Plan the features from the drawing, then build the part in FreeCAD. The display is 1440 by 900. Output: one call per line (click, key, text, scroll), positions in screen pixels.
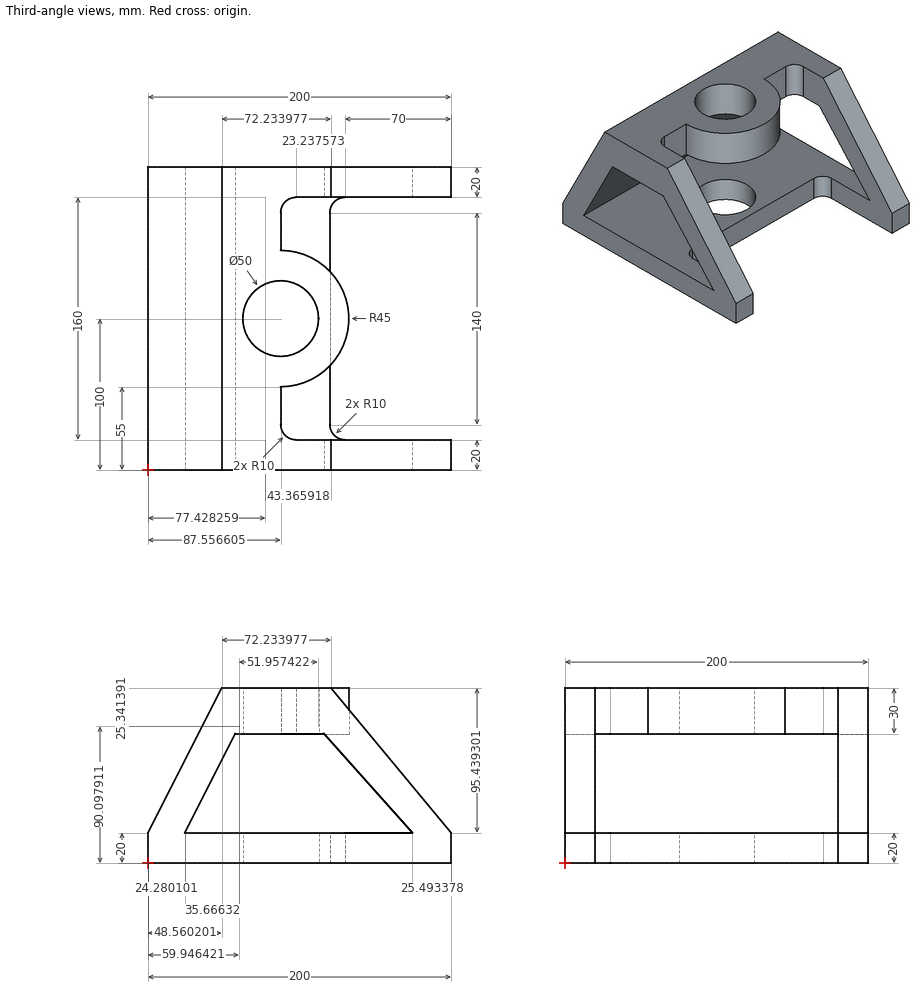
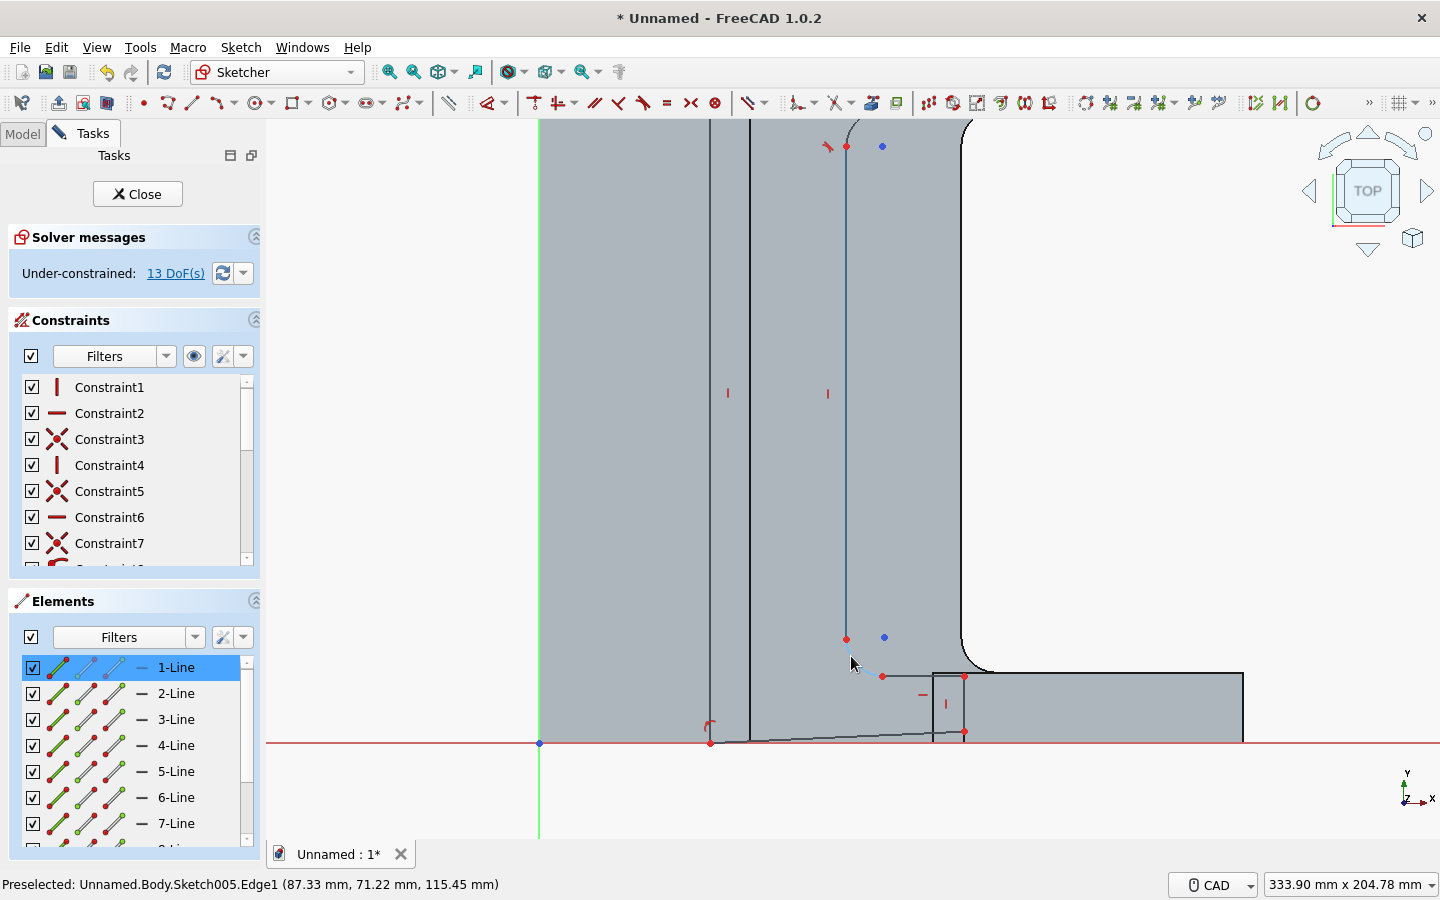
click(851, 655)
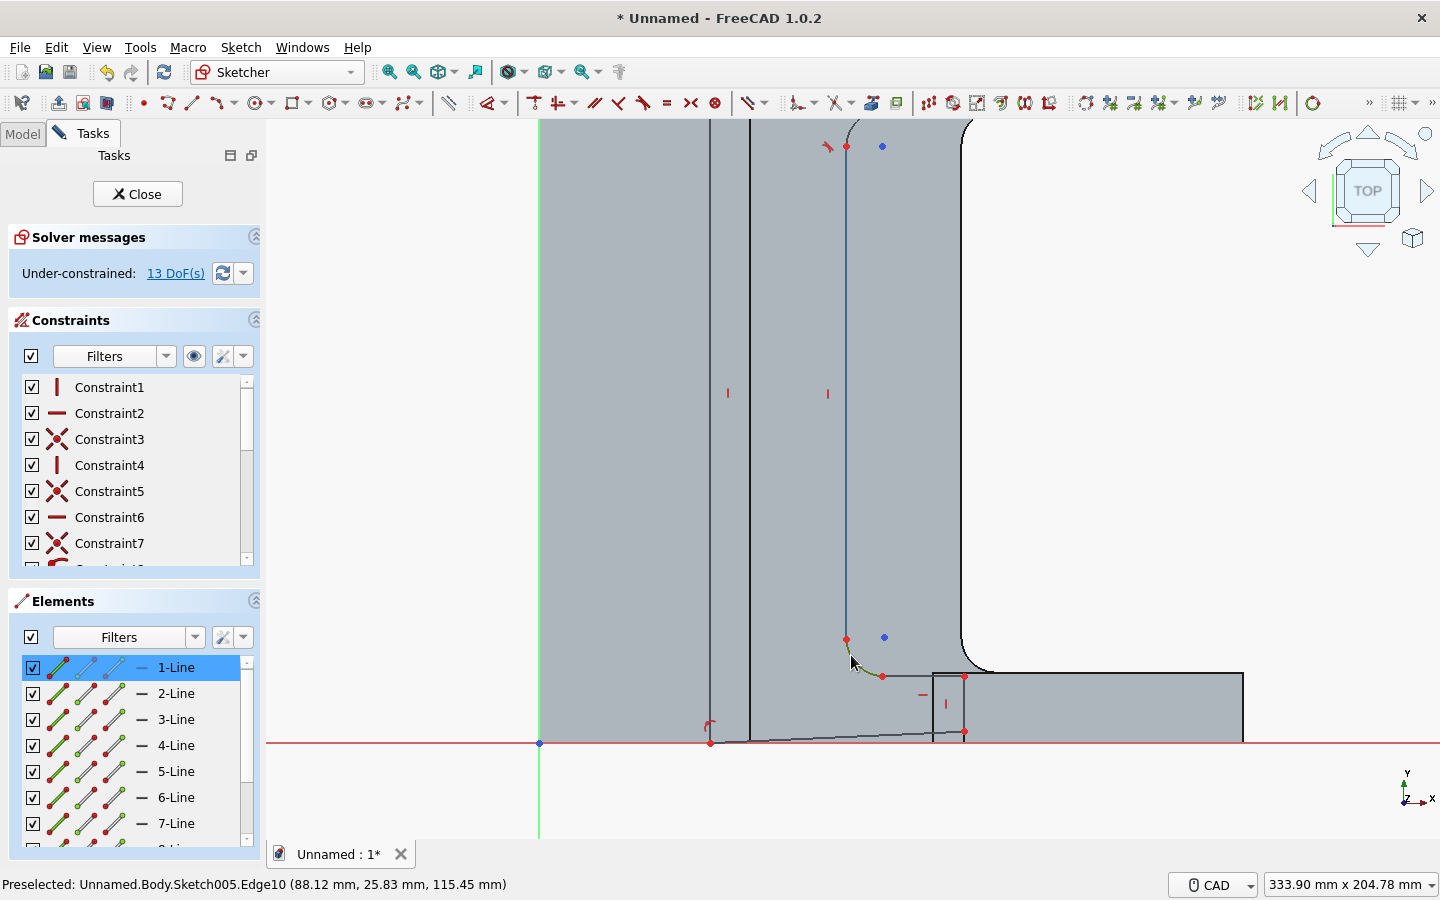
click(644, 104)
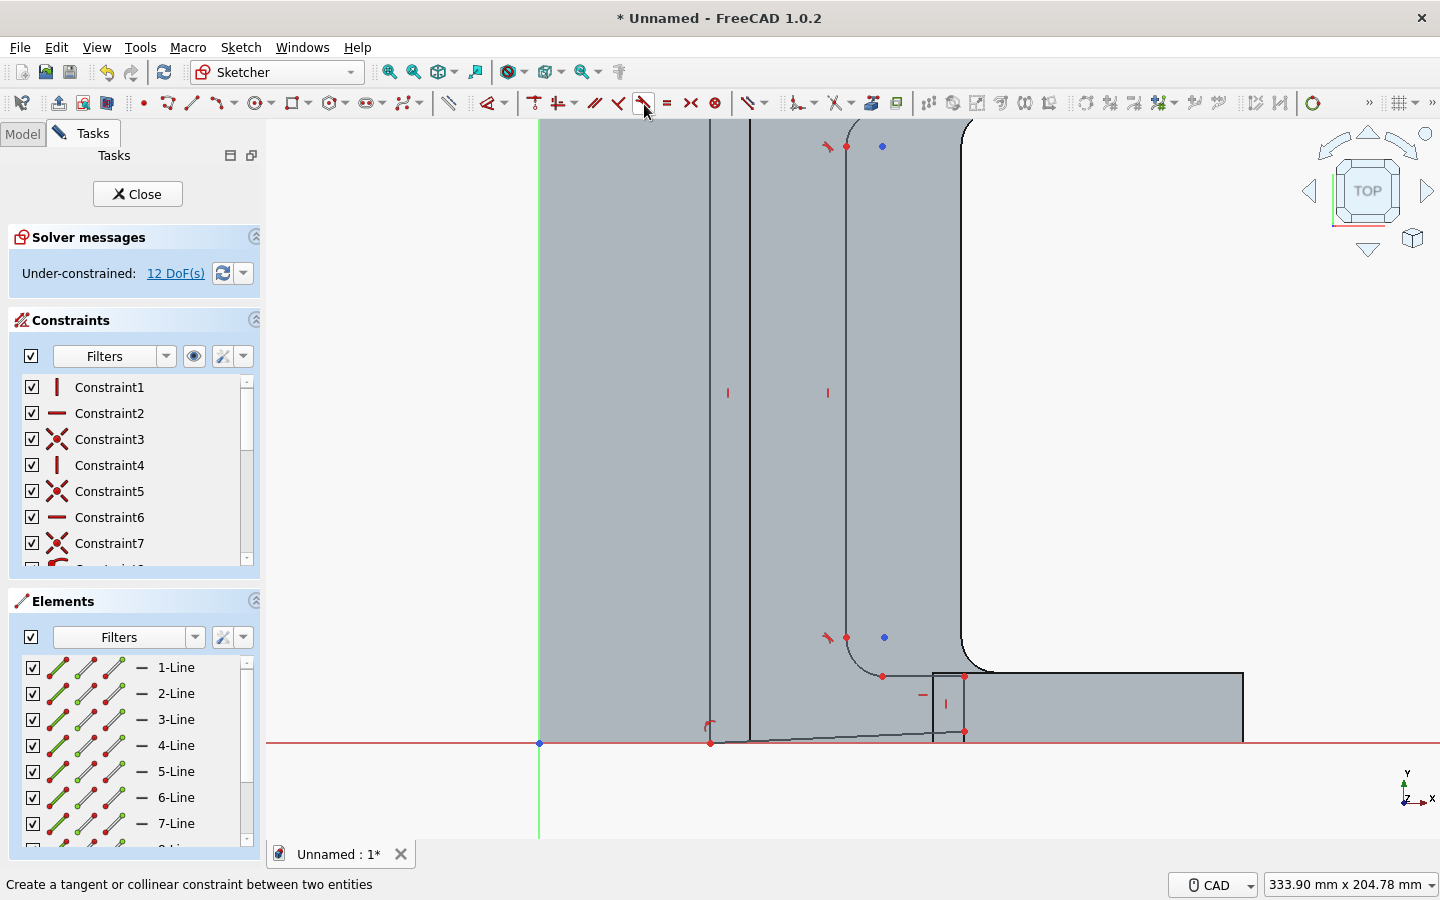
scroll(851, 657, down, 2)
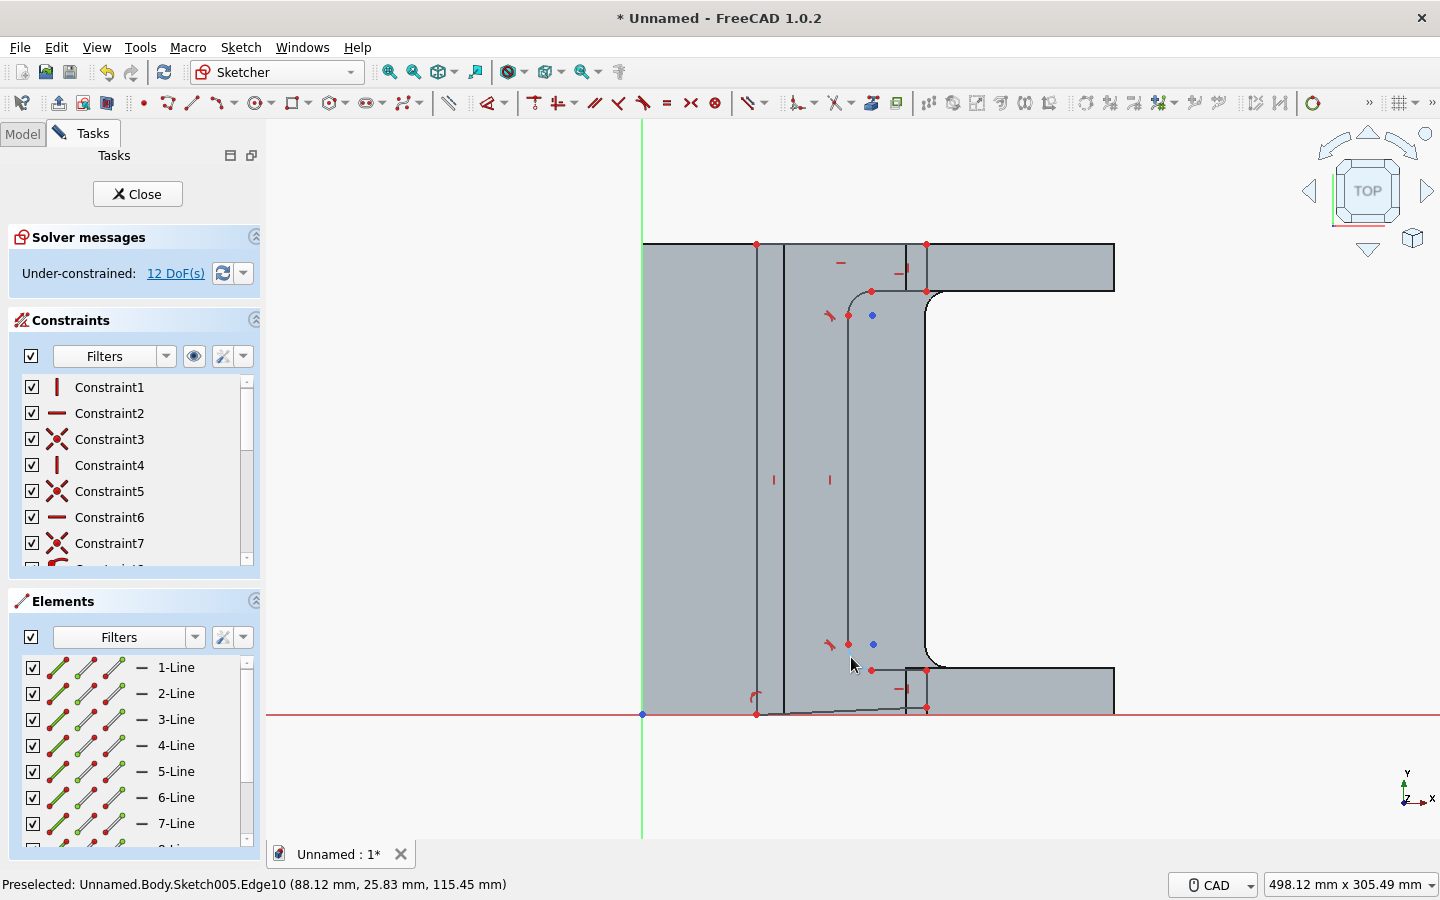
click(888, 291)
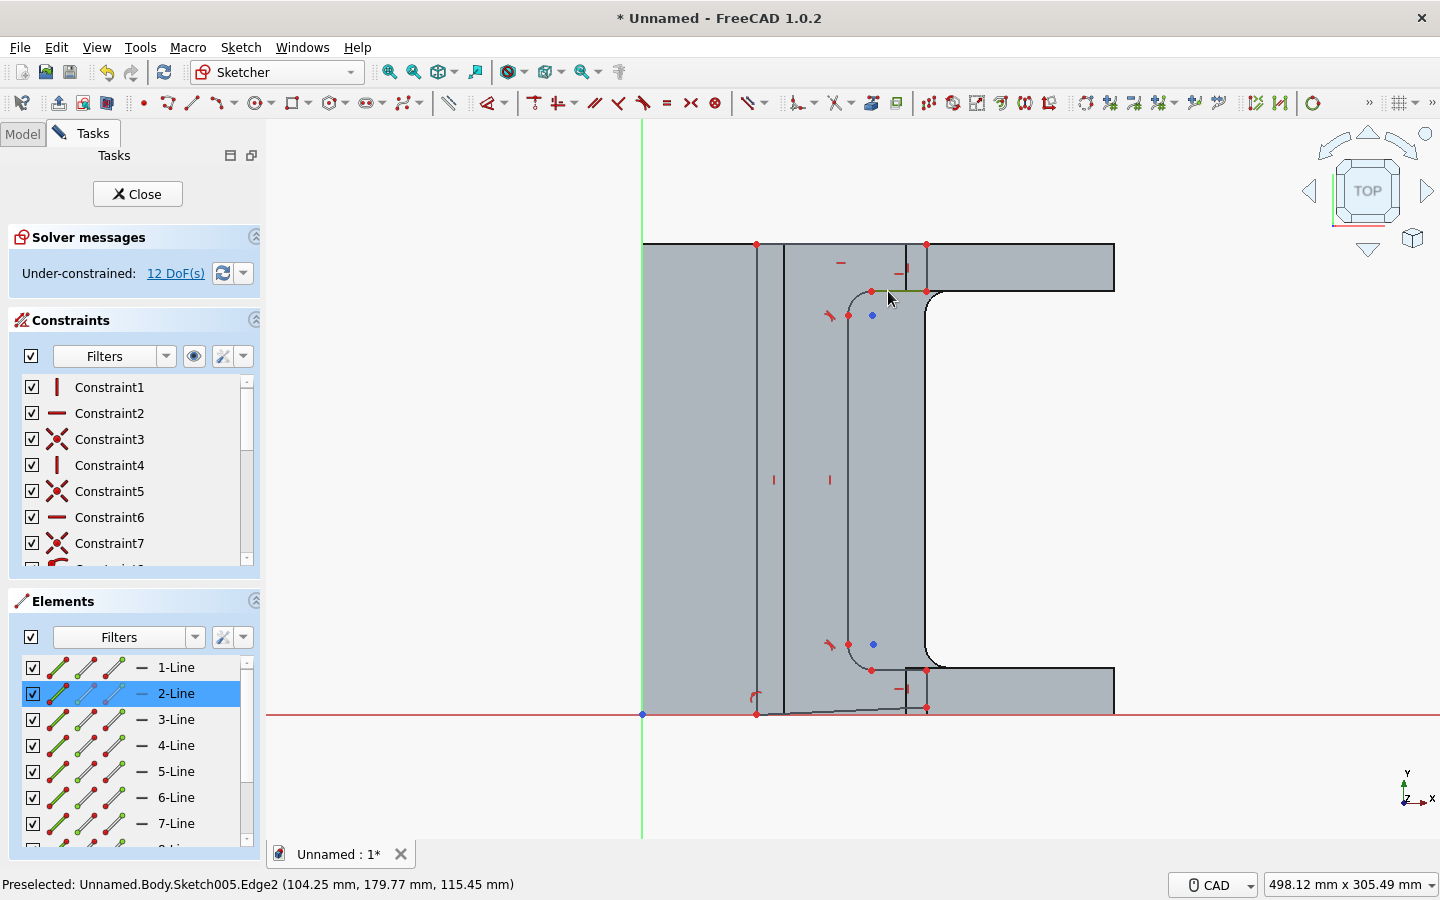
scroll(861, 294, up, 2)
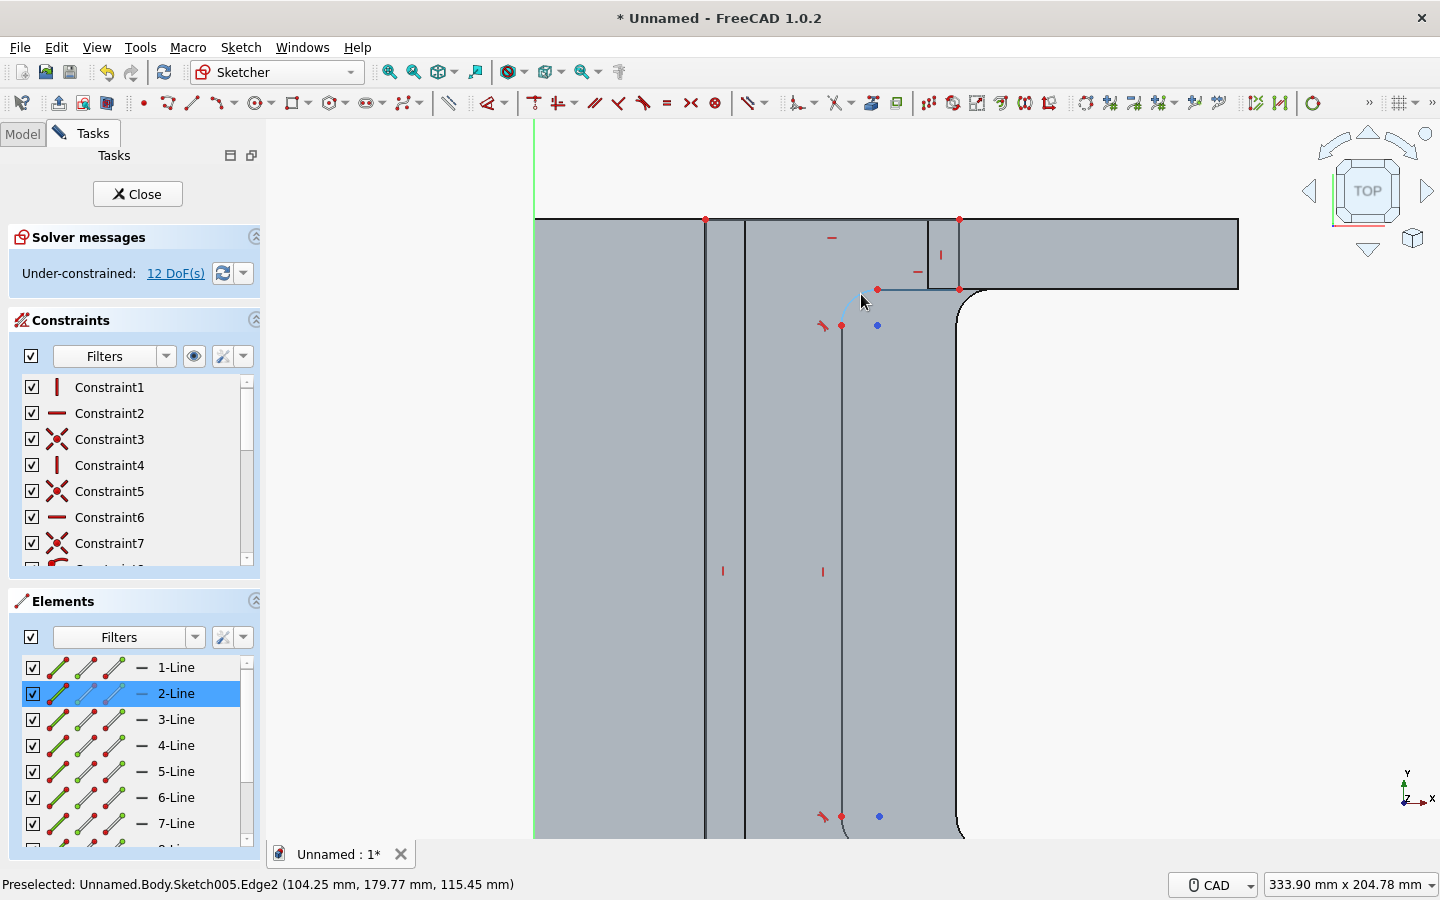
click(861, 294)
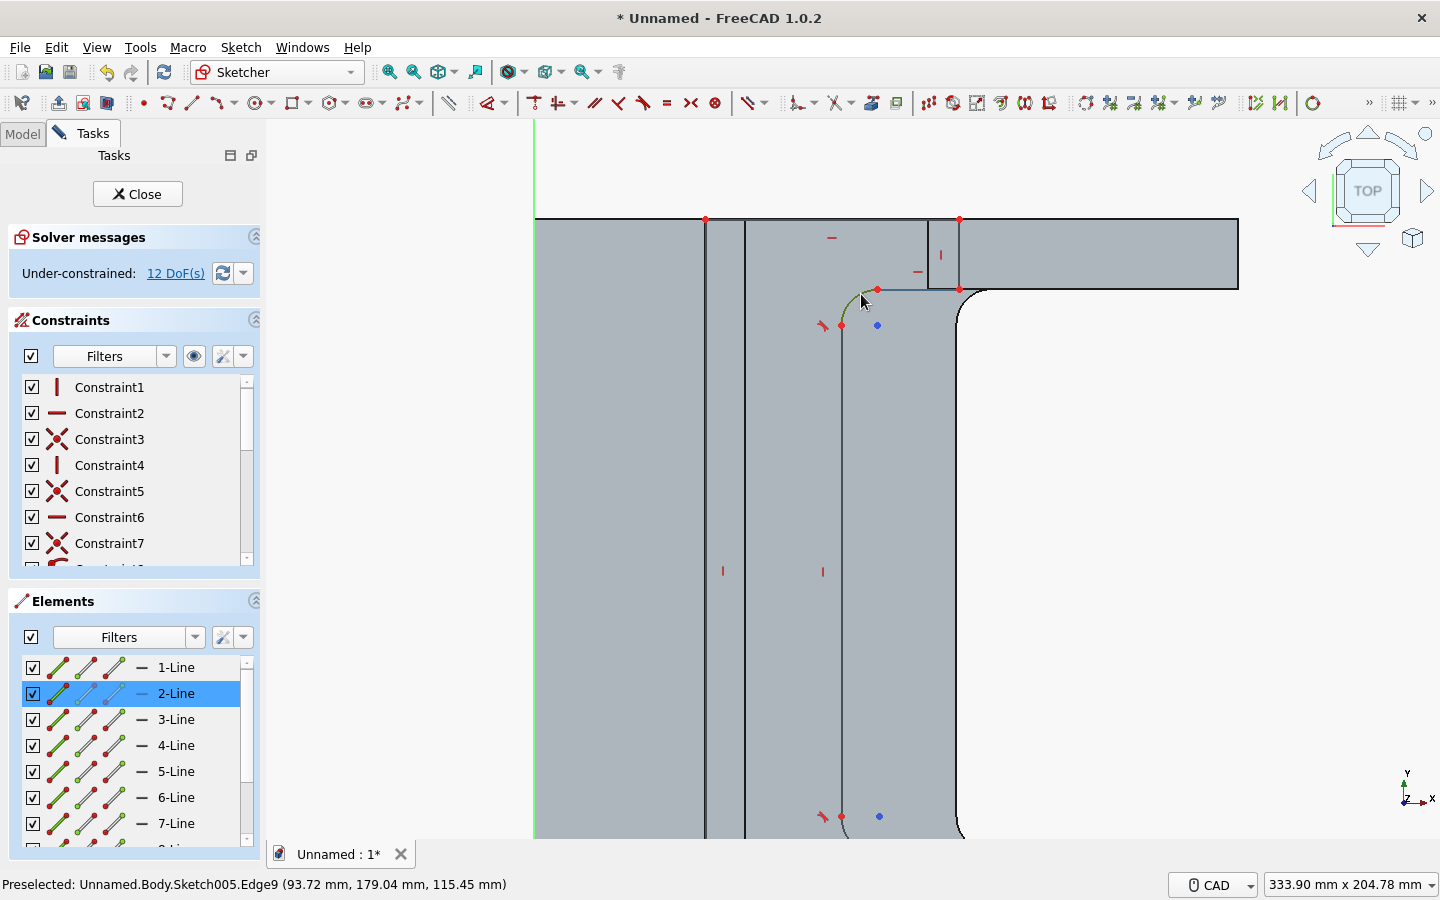
click(644, 104)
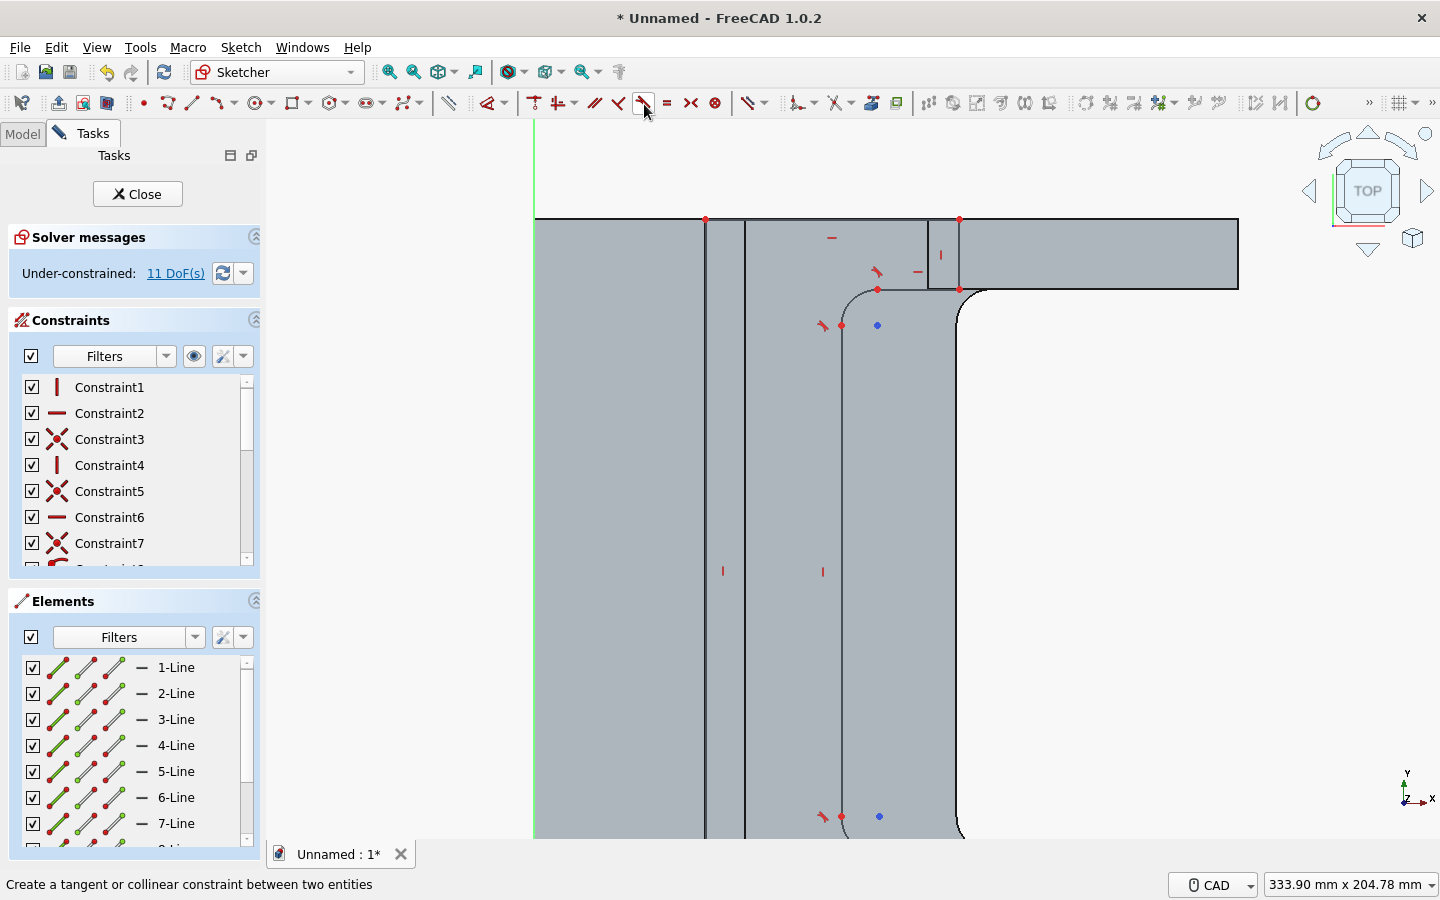
scroll(861, 293, down, 2)